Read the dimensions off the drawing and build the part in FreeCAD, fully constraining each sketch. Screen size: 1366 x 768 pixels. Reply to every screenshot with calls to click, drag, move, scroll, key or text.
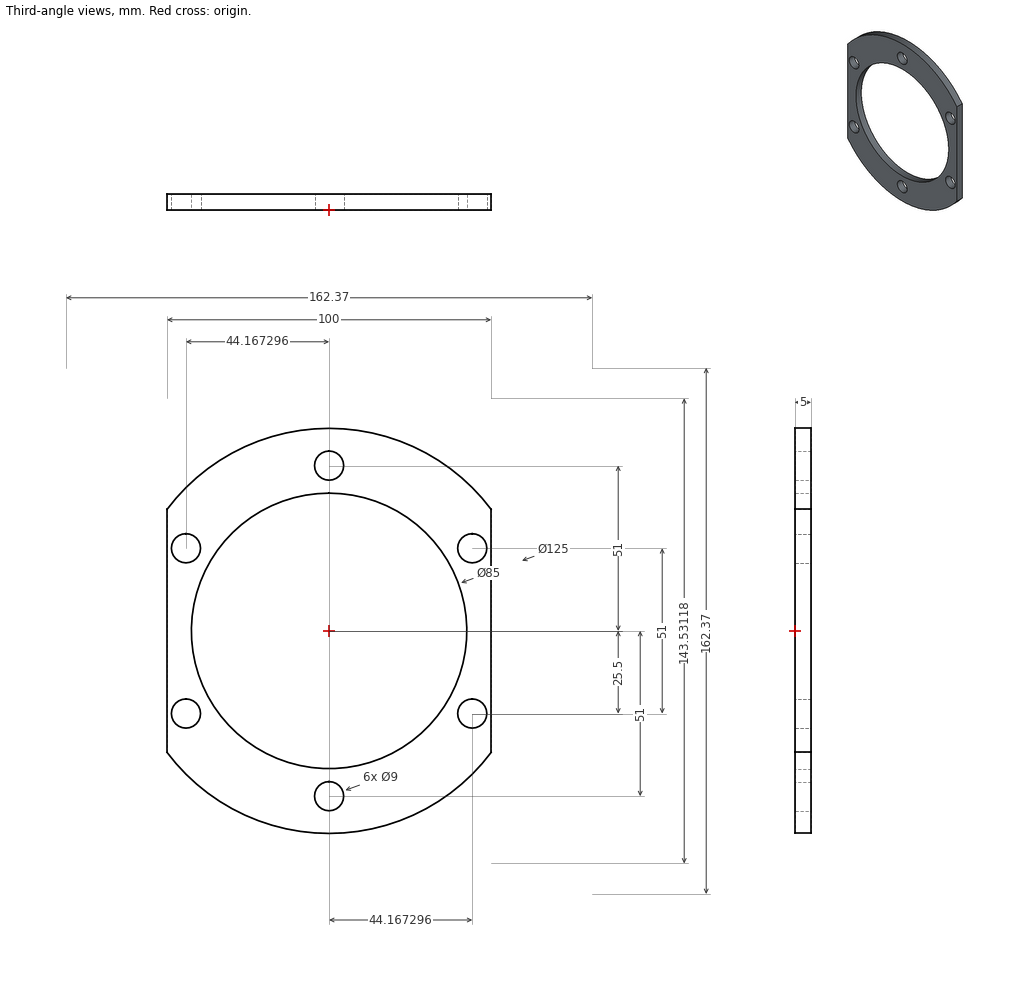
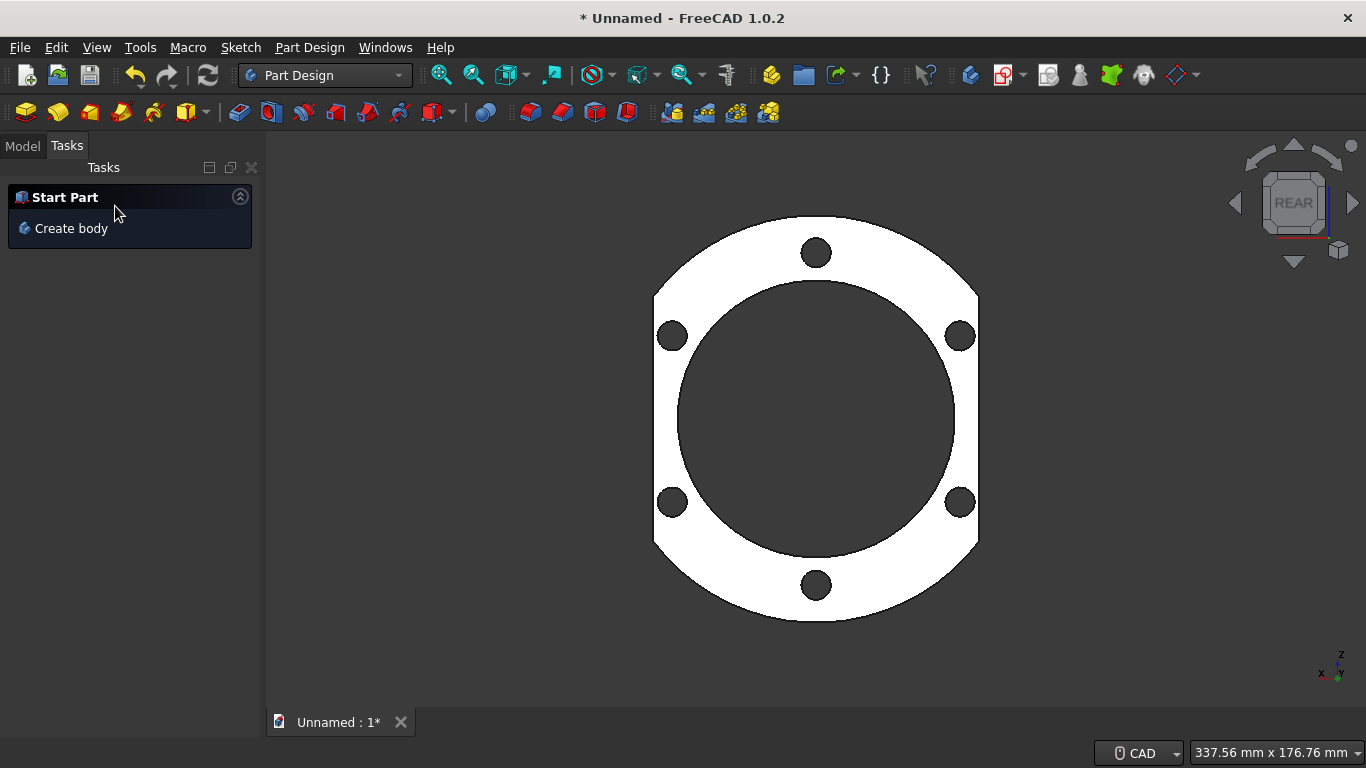
key(0)